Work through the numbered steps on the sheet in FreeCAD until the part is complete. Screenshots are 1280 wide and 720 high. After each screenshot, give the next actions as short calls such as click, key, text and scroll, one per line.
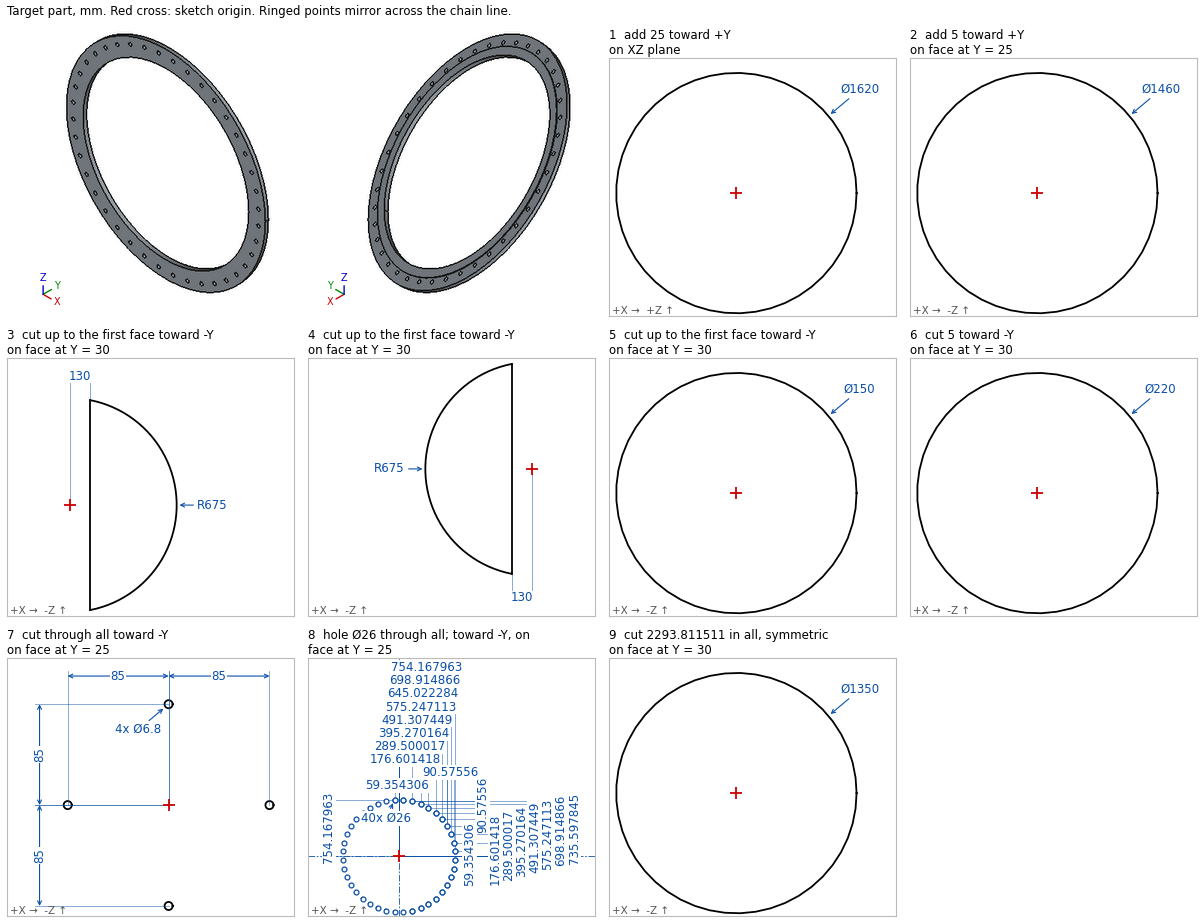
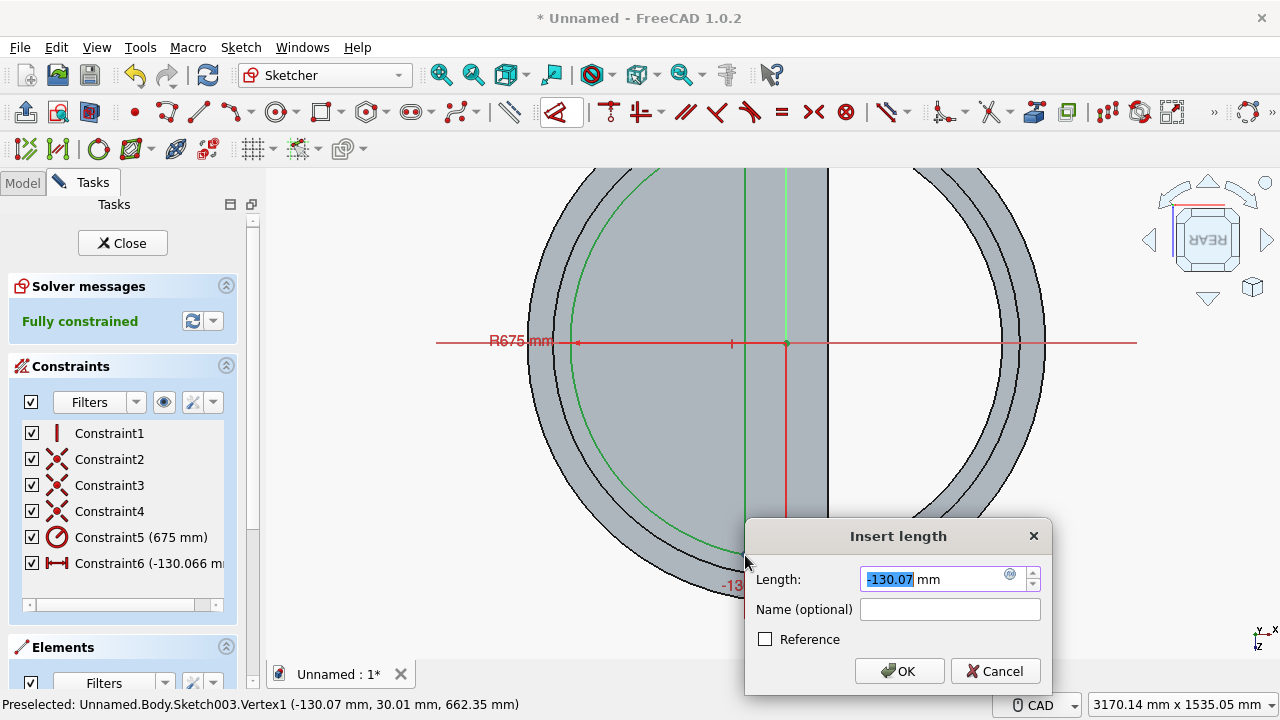
text(-130)
key(Return)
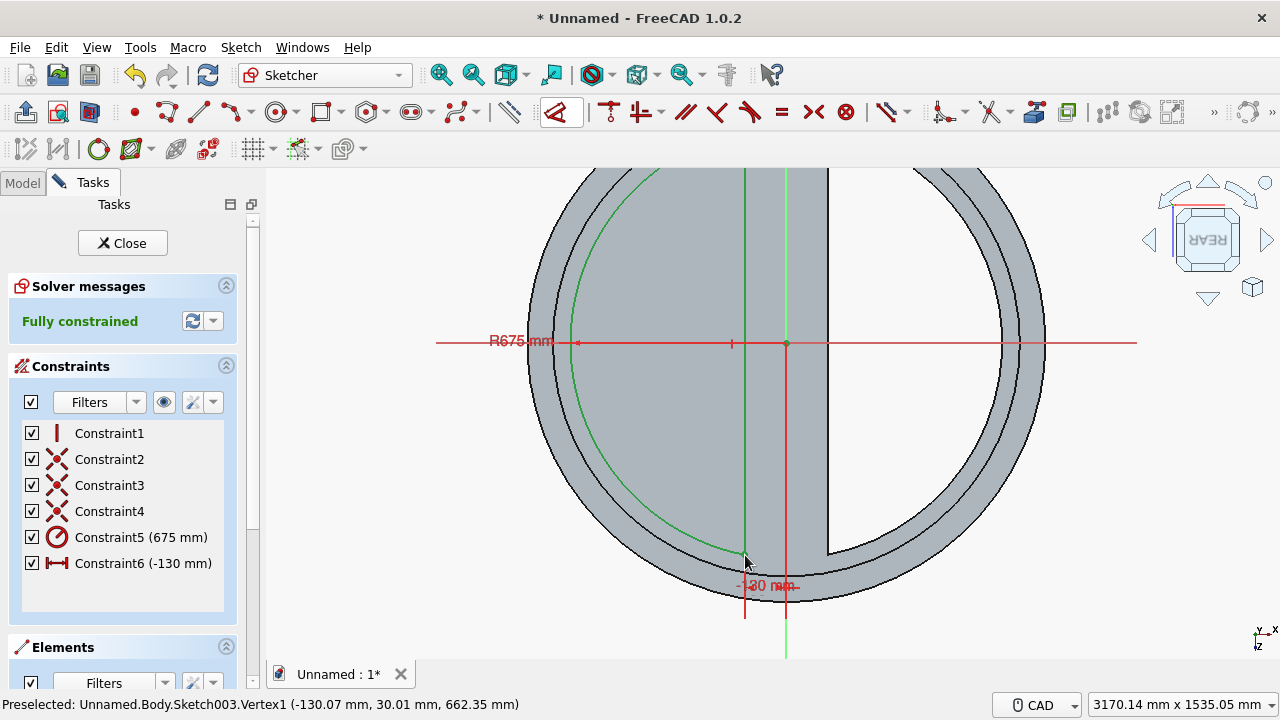
click(123, 243)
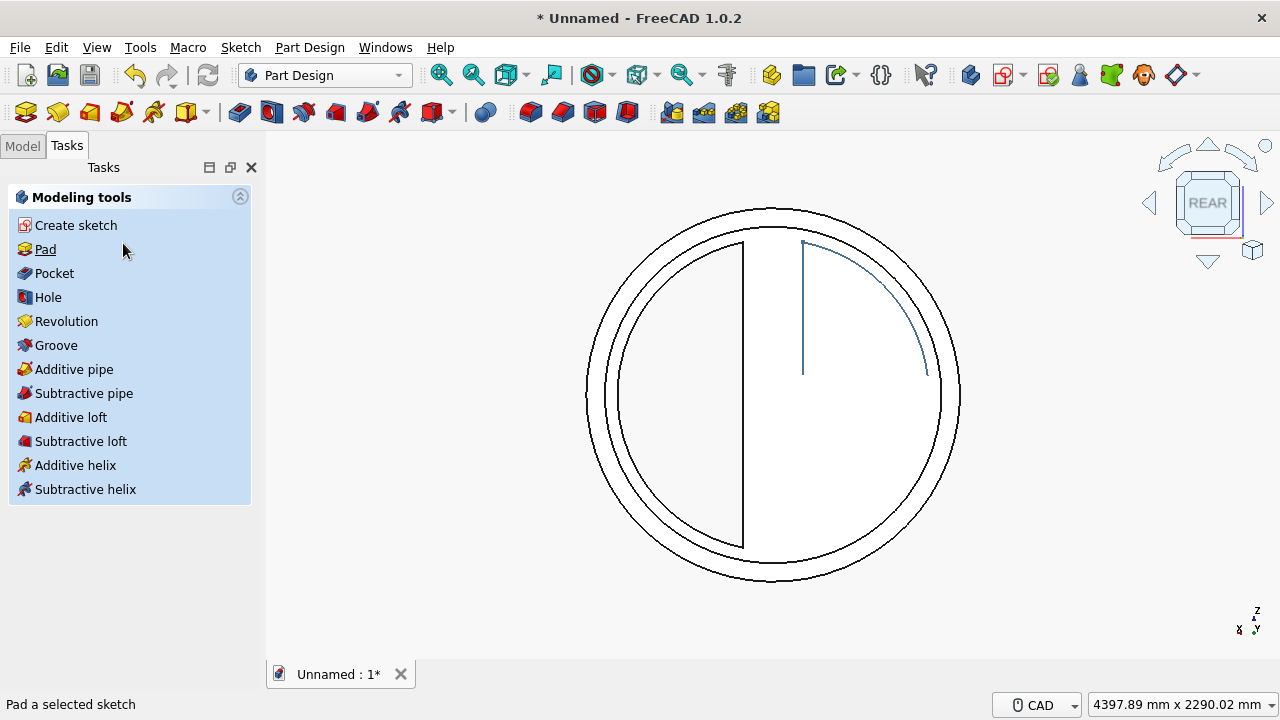
click(240, 112)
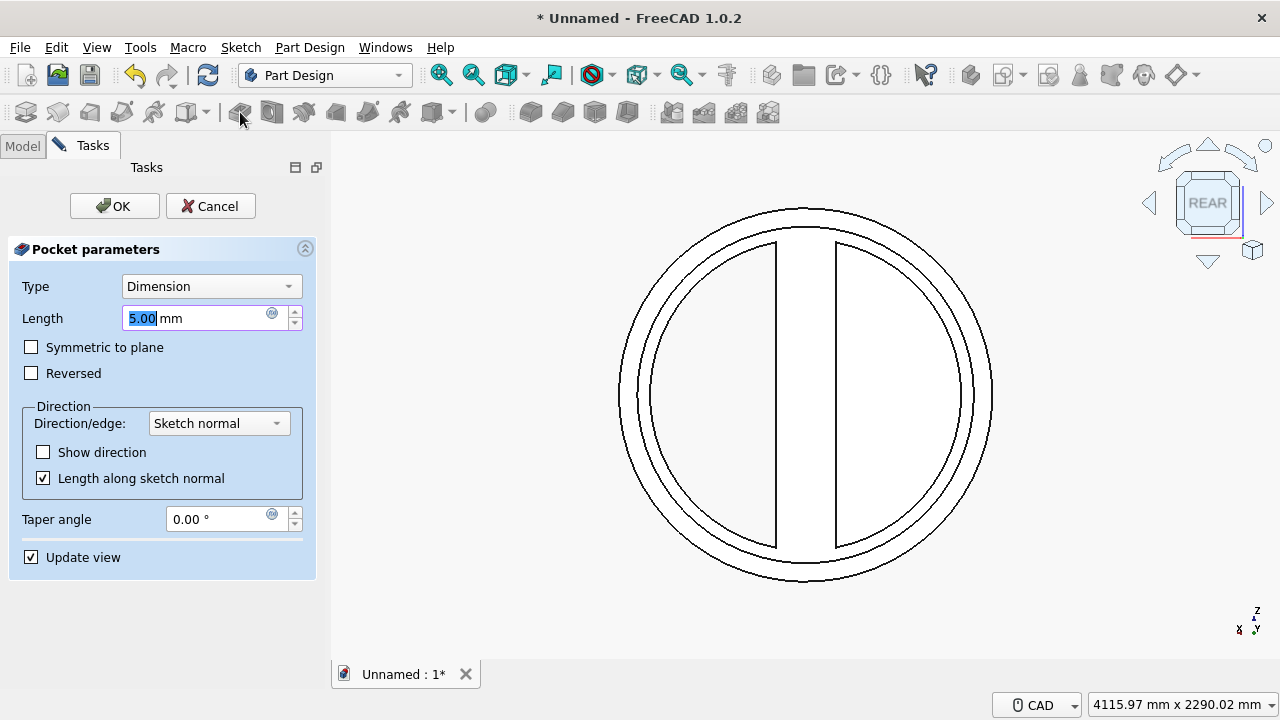
click(212, 286)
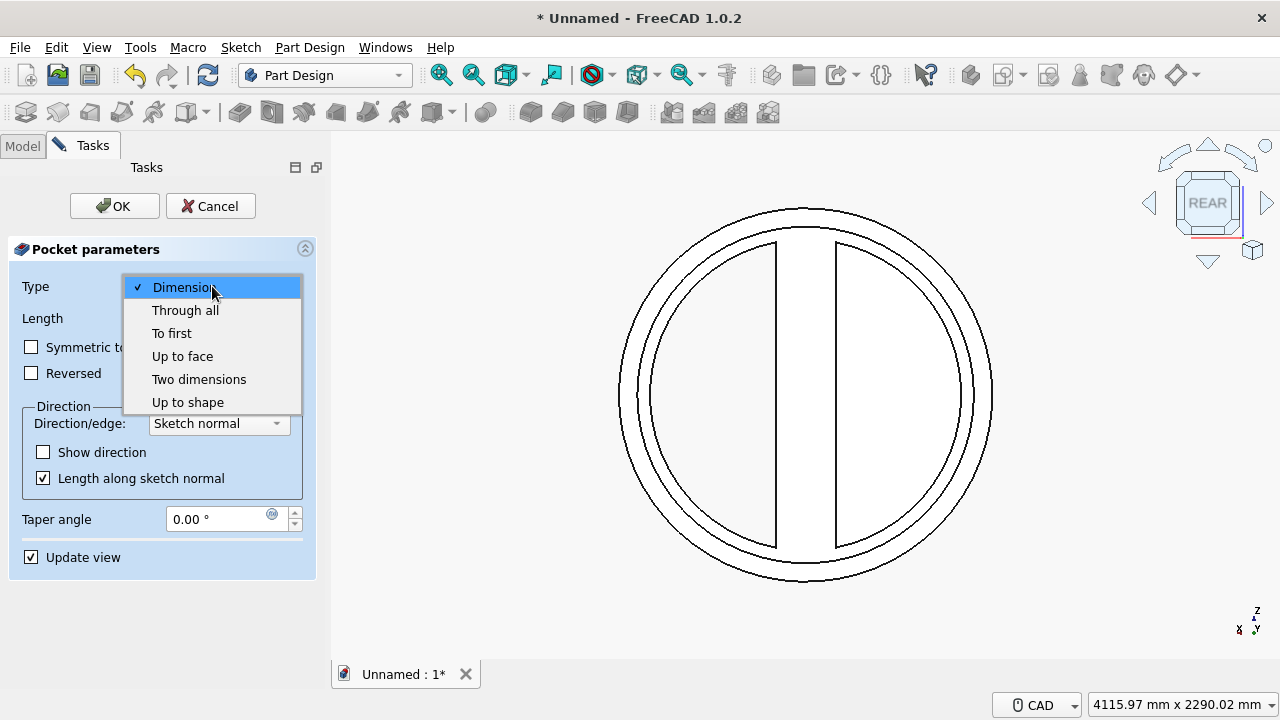
click(212, 334)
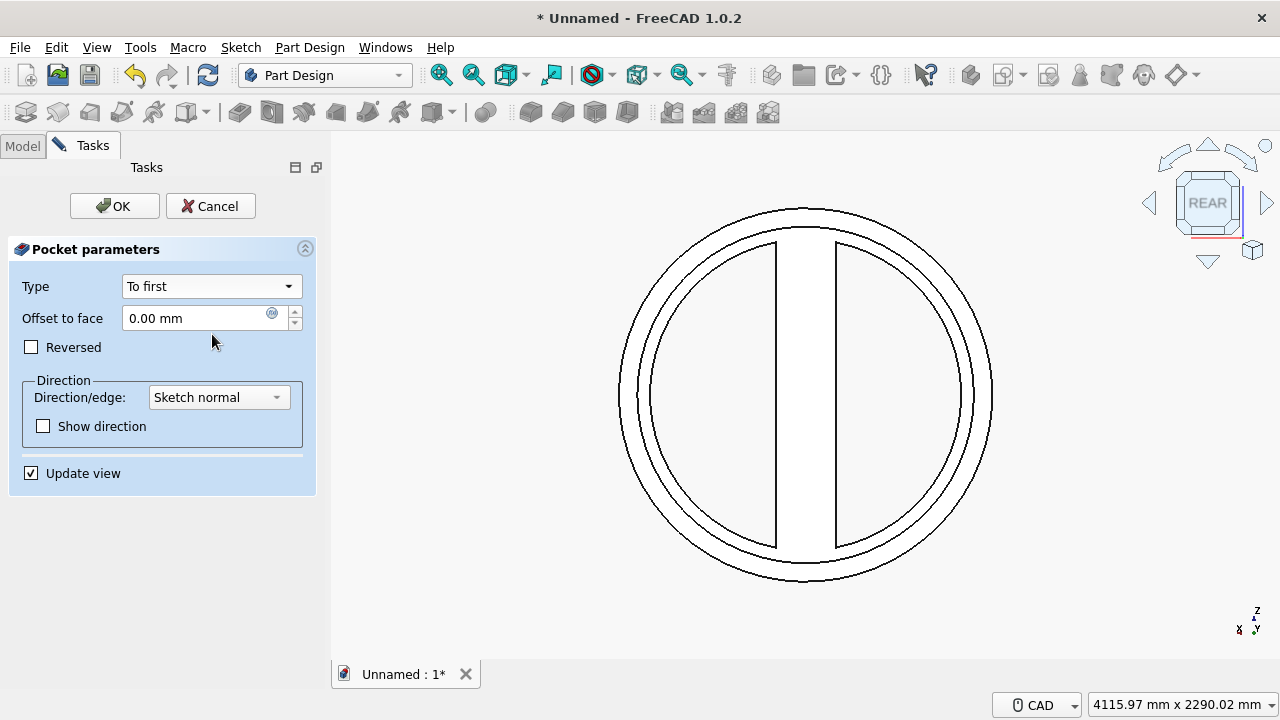
click(115, 206)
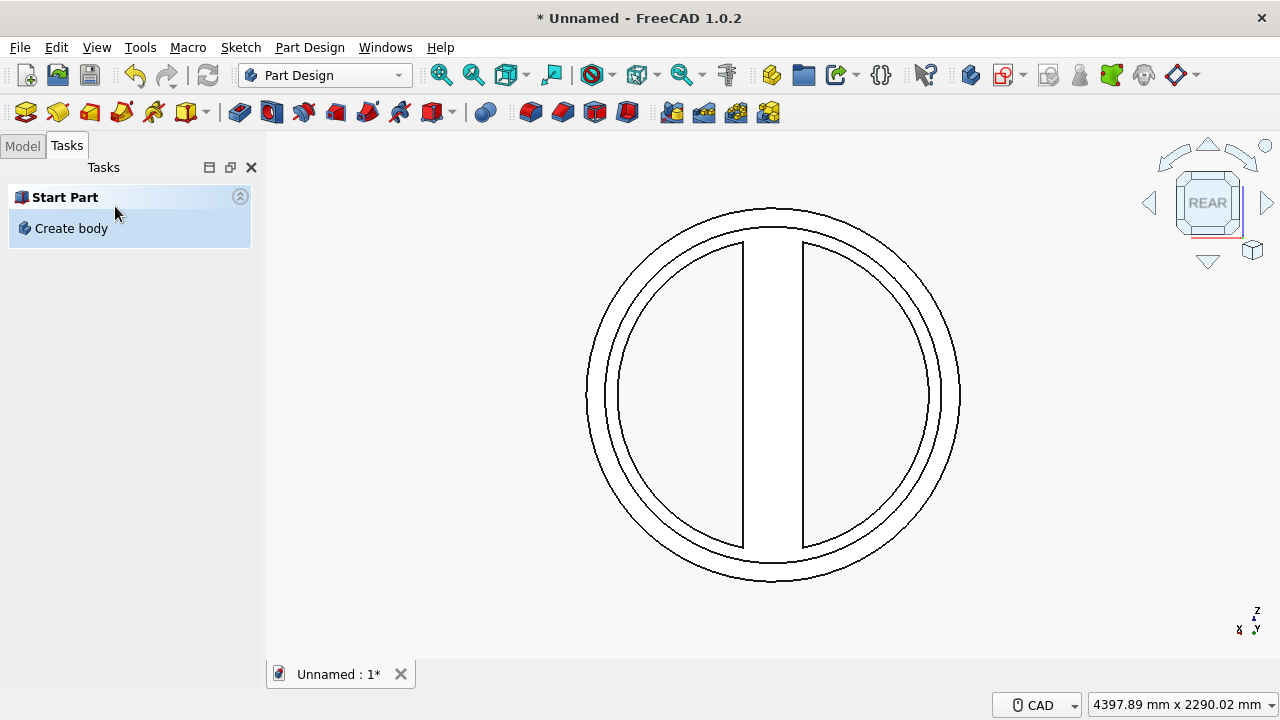
click(773, 490)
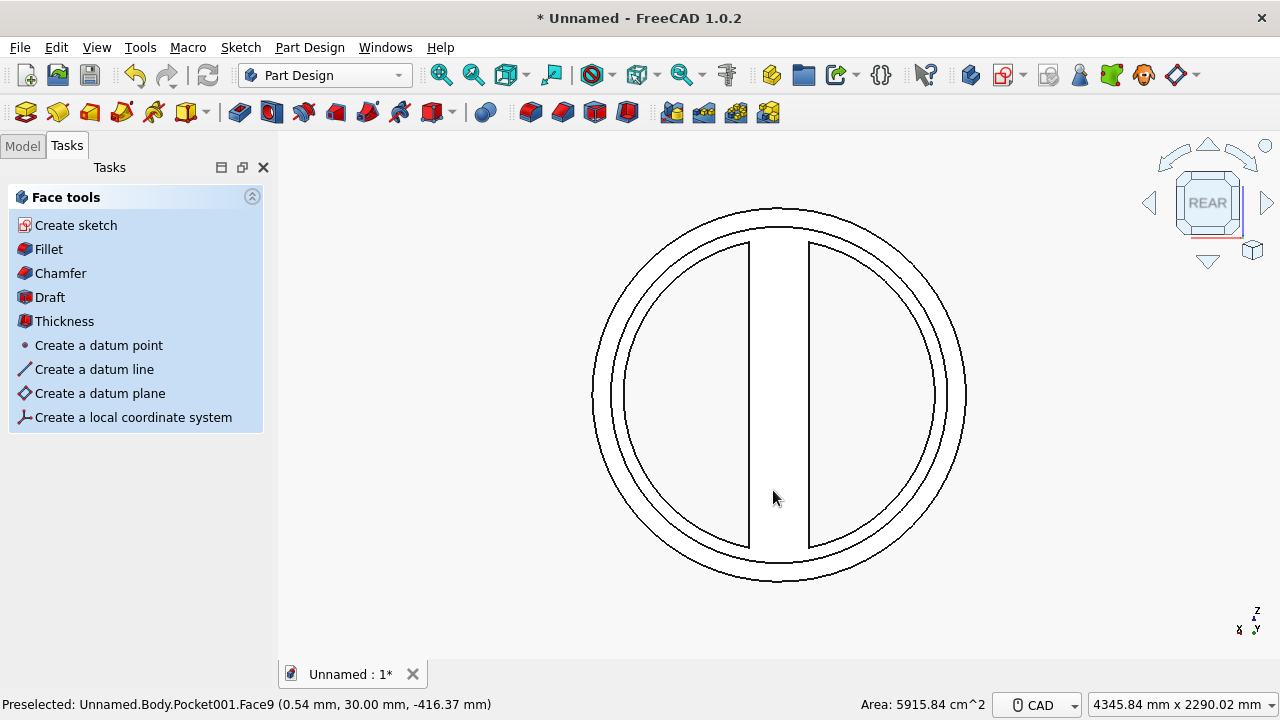
click(1004, 76)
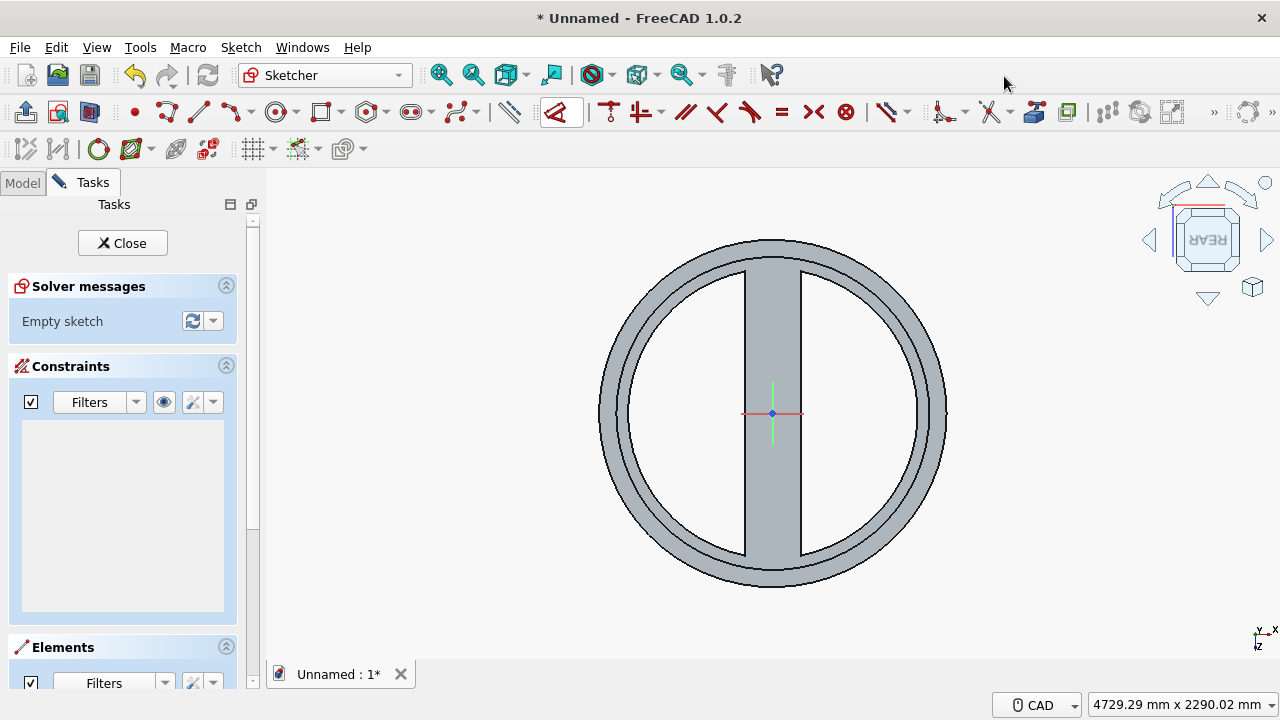
scroll(781, 413, up, 11)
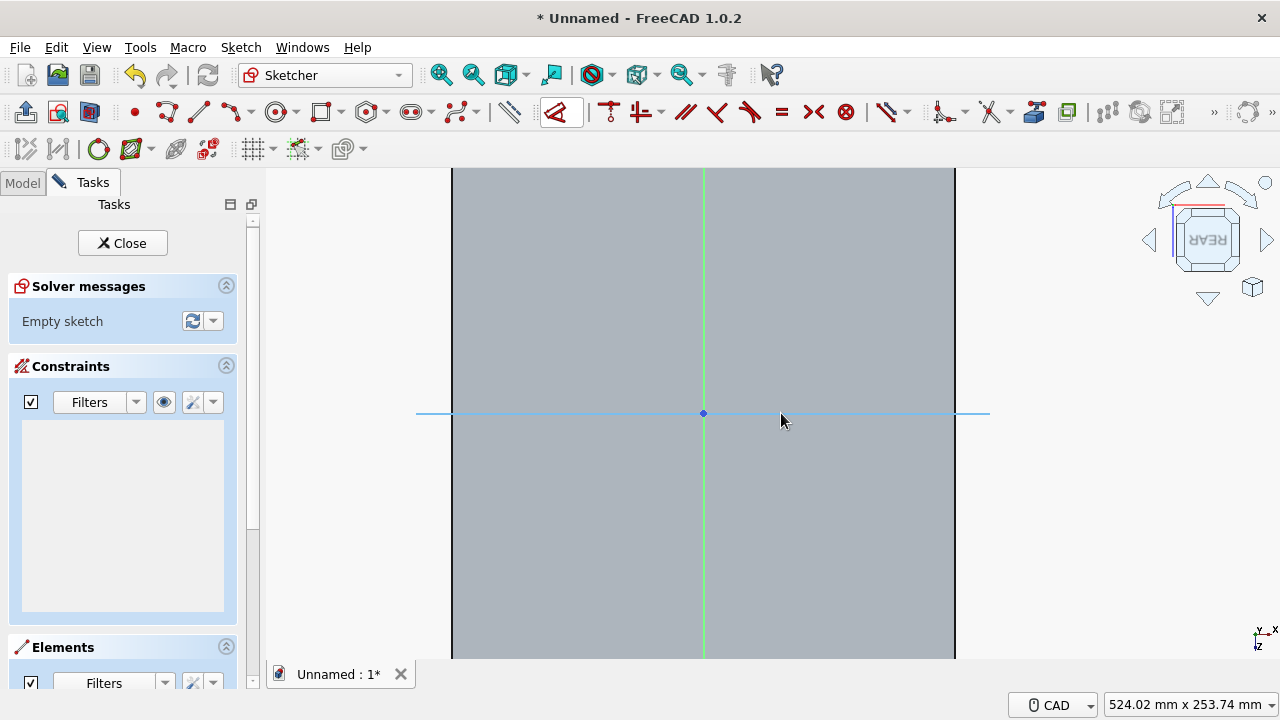
click(276, 112)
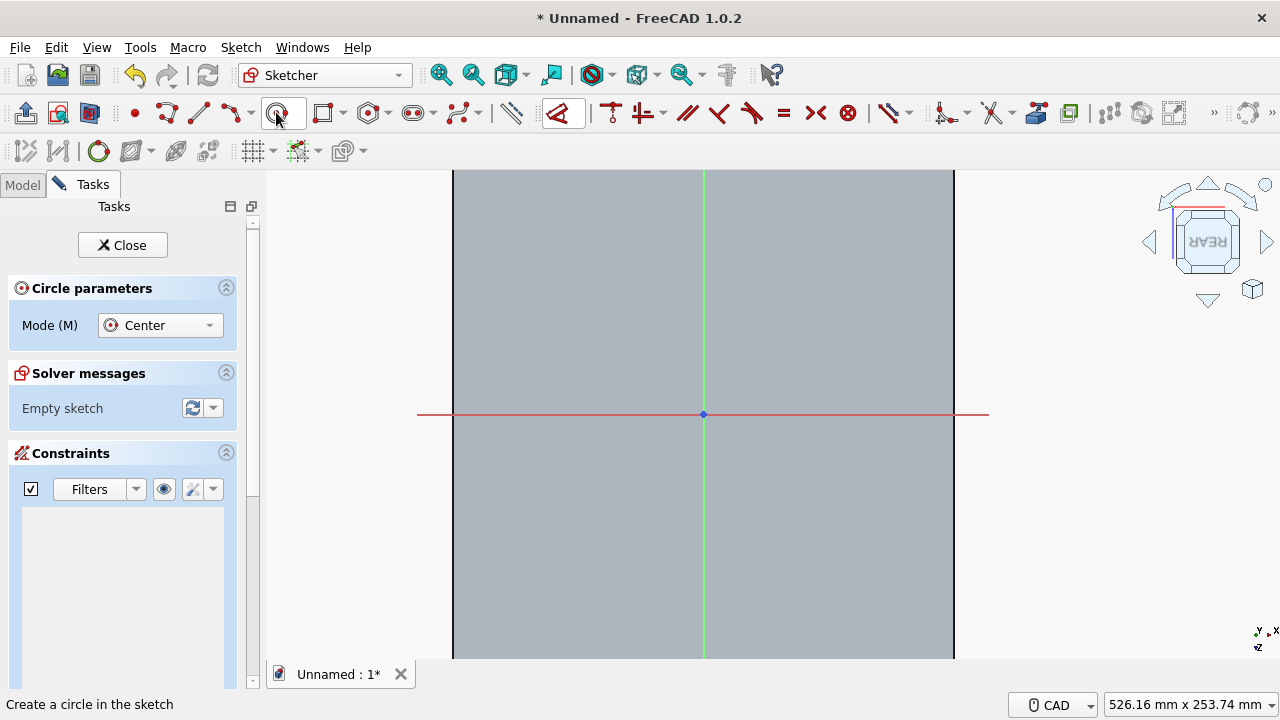
click(704, 414)
click(806, 312)
key(Escape)